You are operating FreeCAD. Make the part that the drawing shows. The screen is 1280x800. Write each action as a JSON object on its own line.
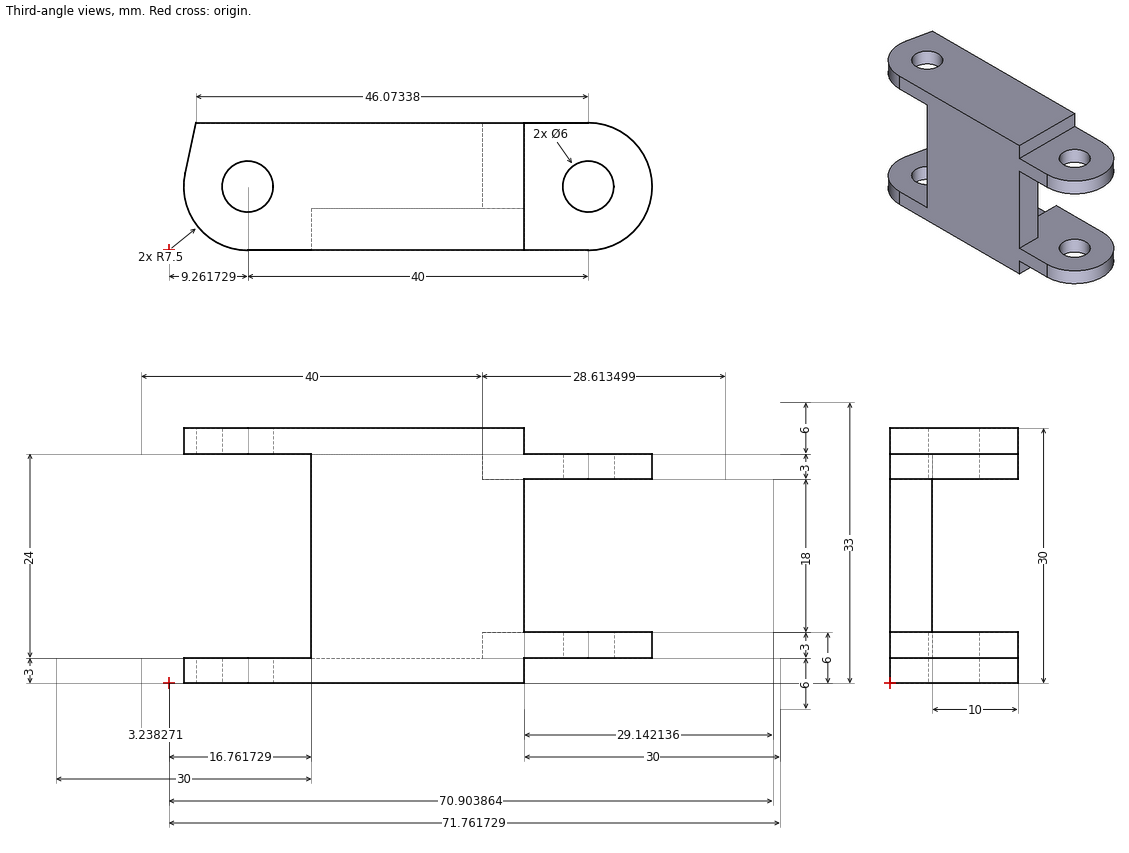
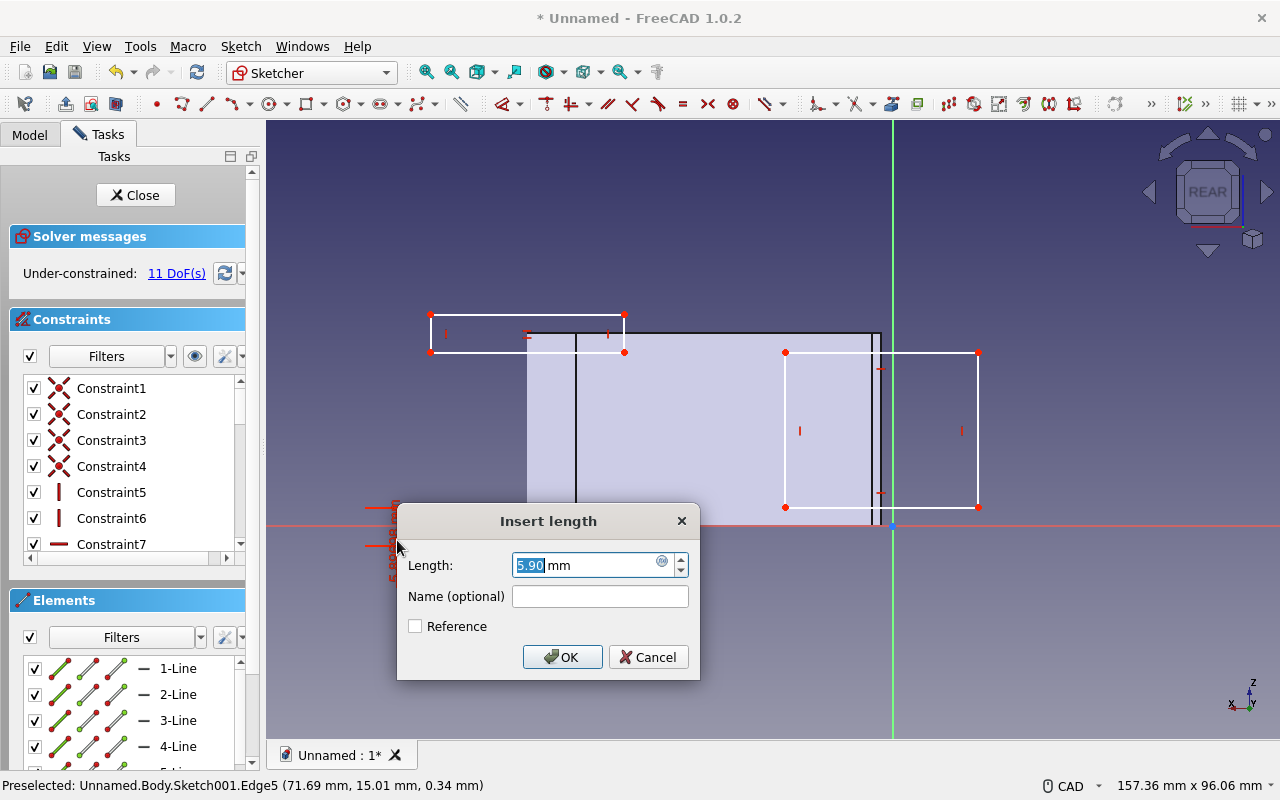
{"action": "type", "text": "6"}
{"action": "key", "text": "Return"}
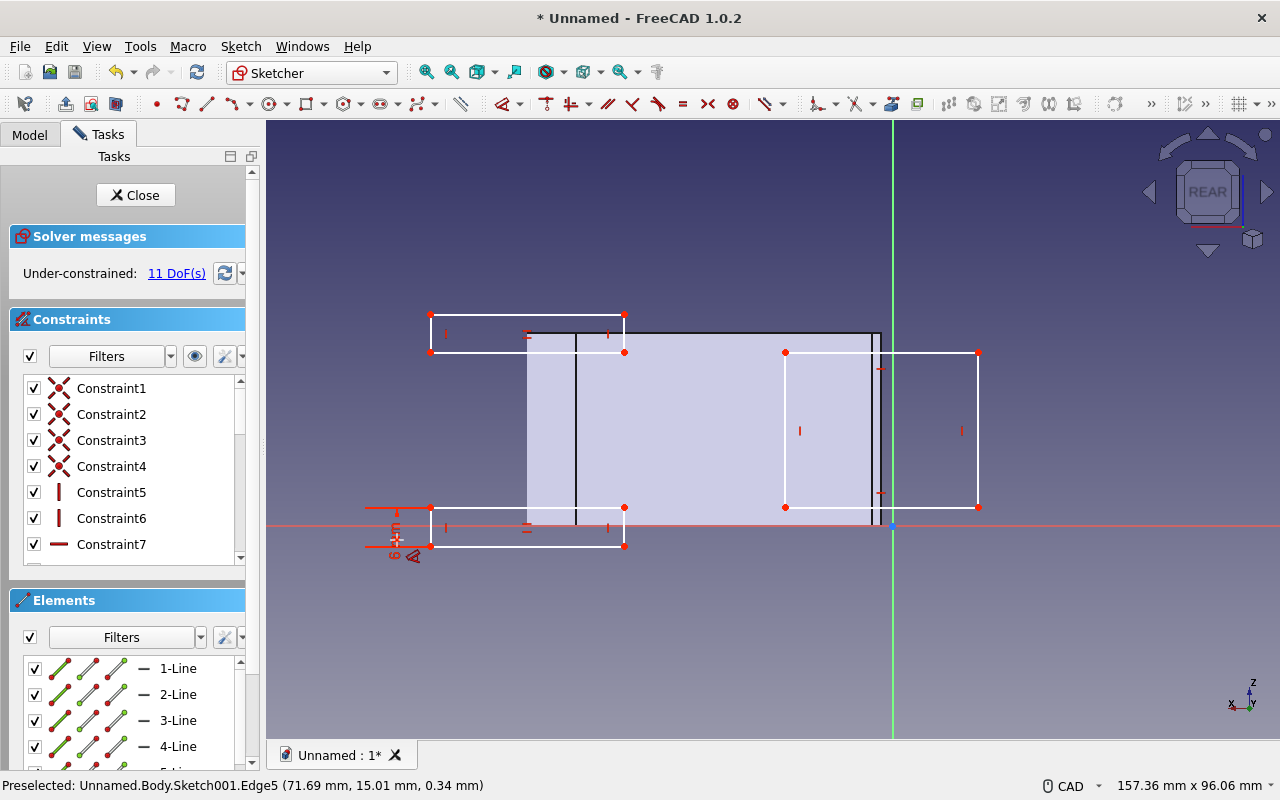
{"action": "left_click", "coordinate": [431, 326]}
{"action": "left_click", "coordinate": [397, 334]}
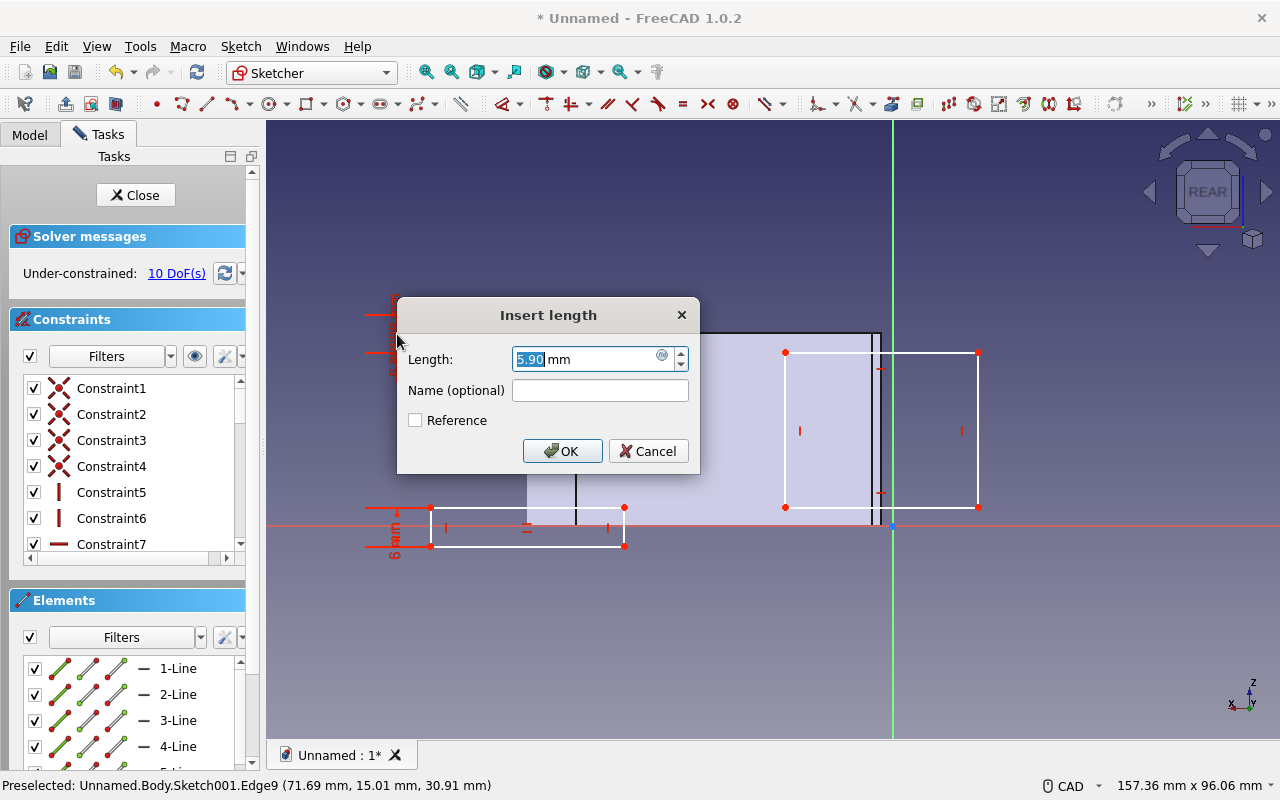
{"action": "type", "text": "6"}
{"action": "key", "text": "Return"}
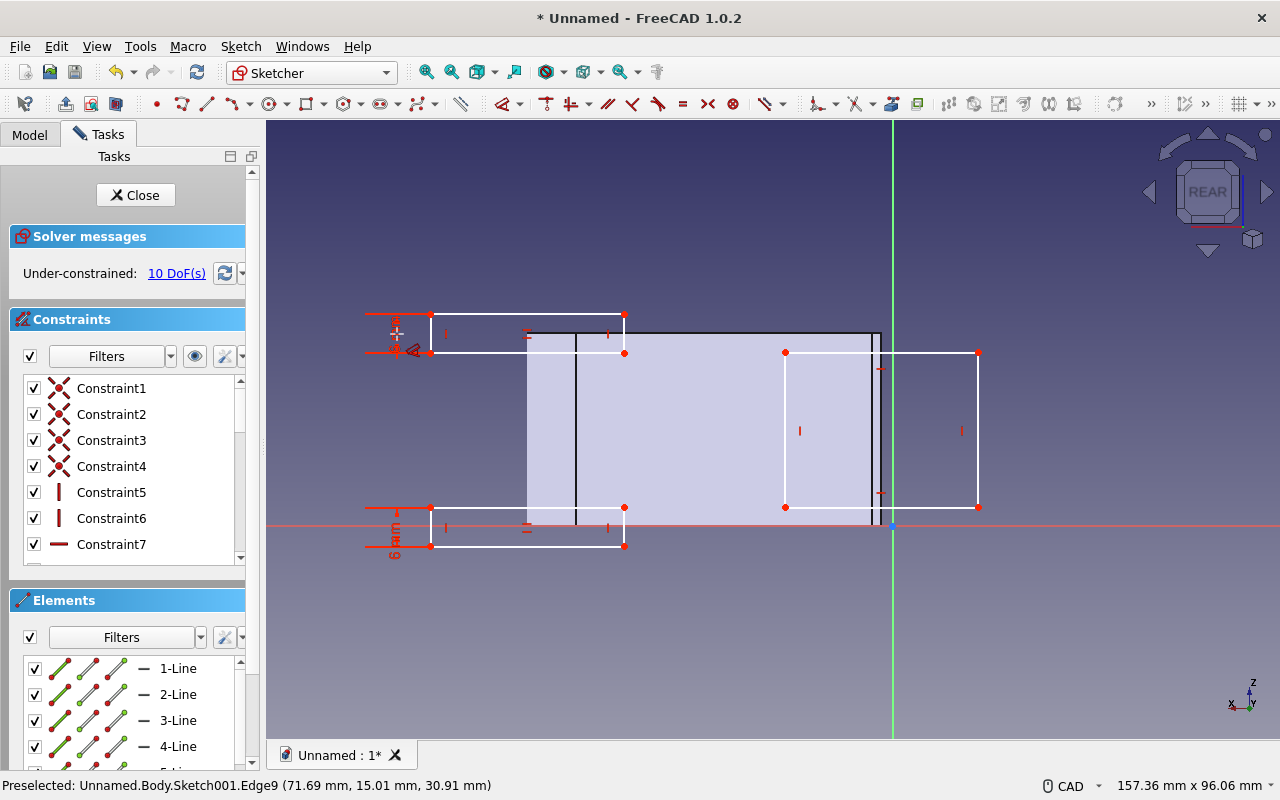
{"action": "left_click", "coordinate": [785, 399]}
{"action": "left_click", "coordinate": [819, 430]}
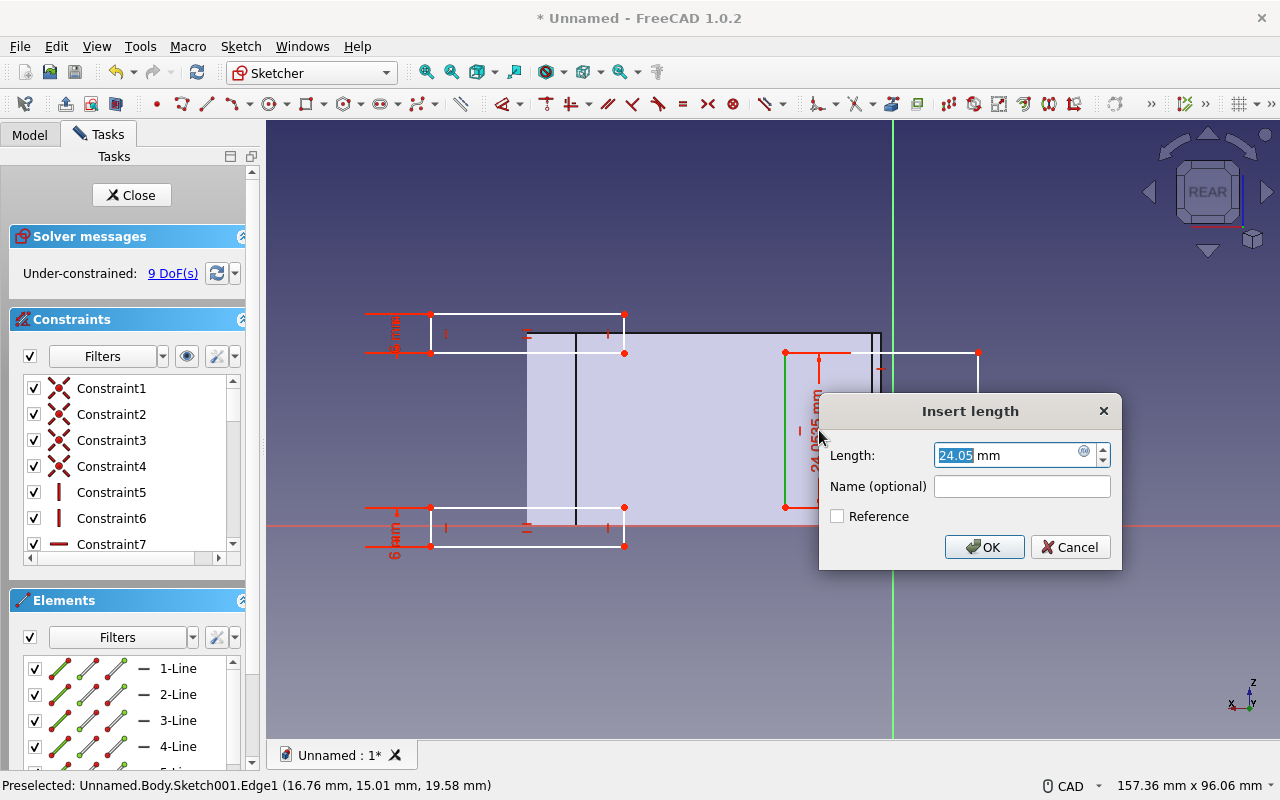
{"action": "type", "text": "24"}
{"action": "key", "text": "Return"}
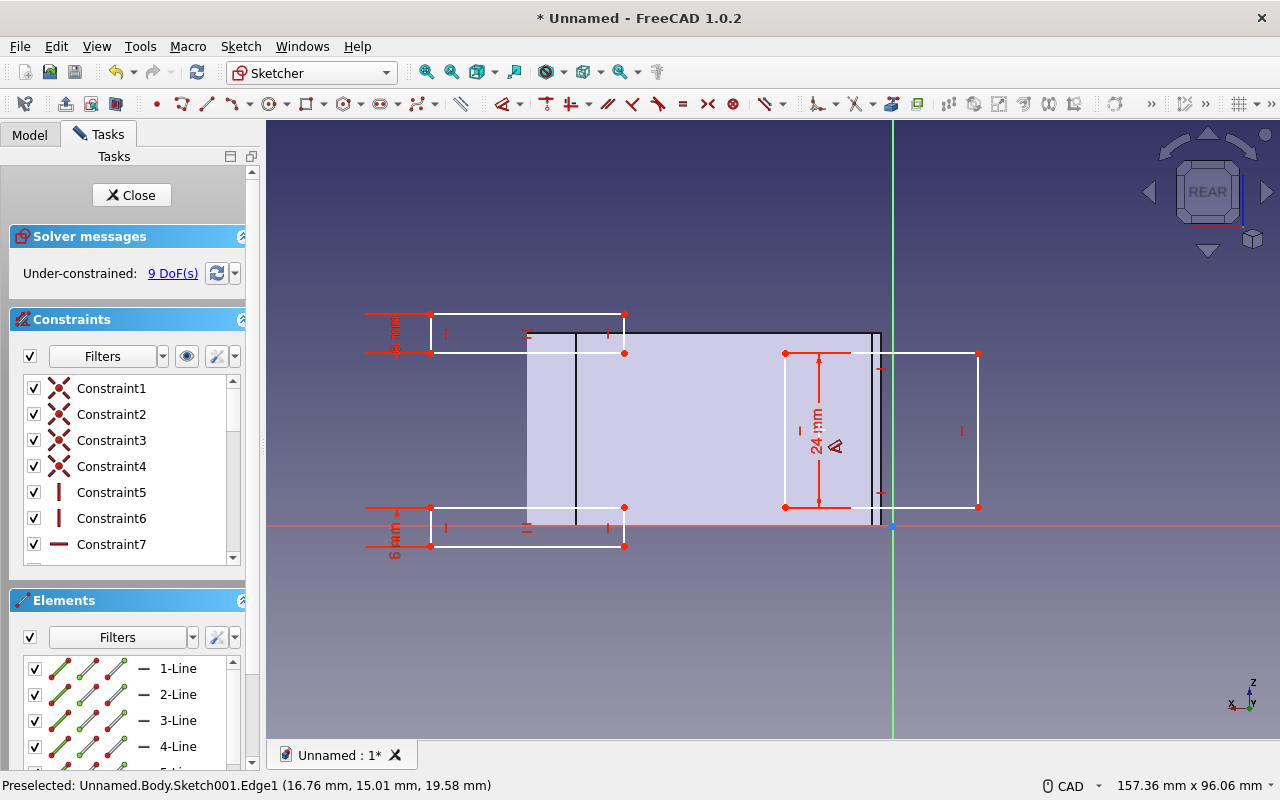
{"action": "left_click", "coordinate": [843, 508]}
{"action": "left_click", "coordinate": [837, 542]}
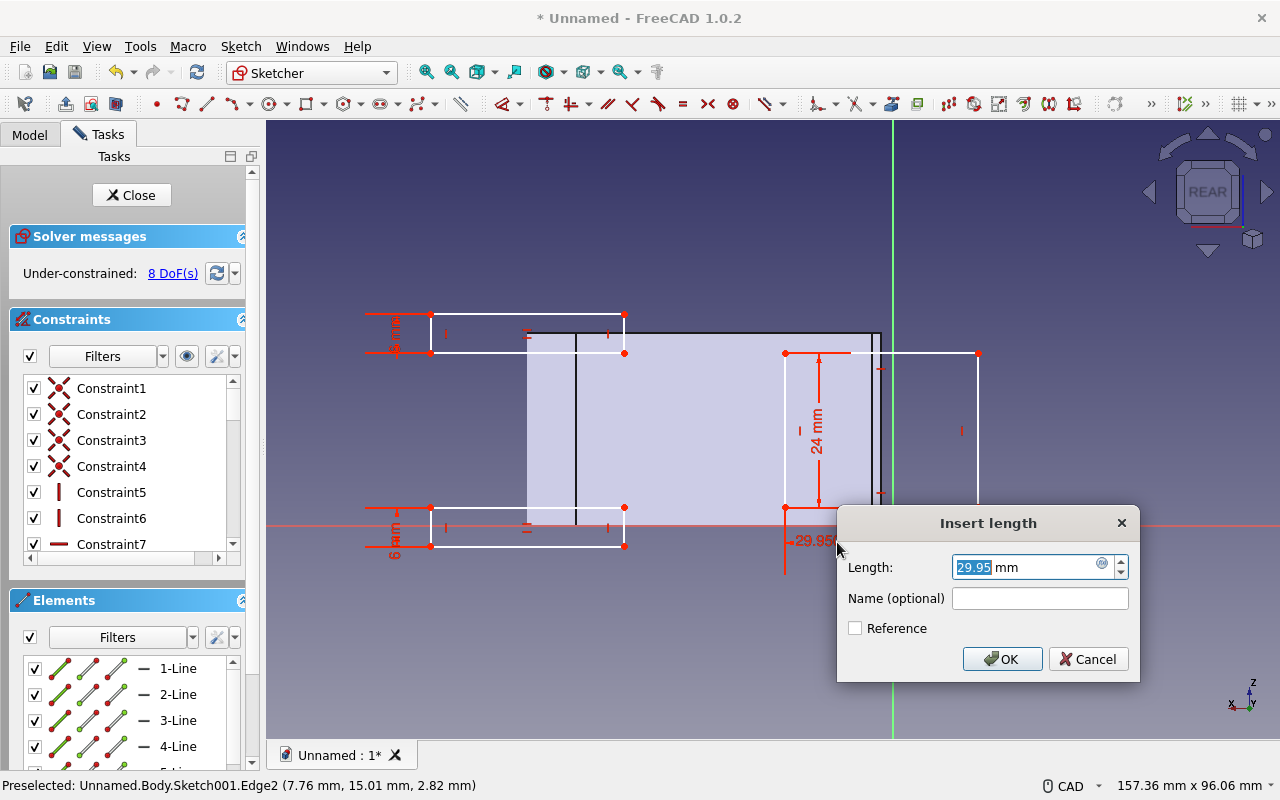
{"action": "type", "text": "30"}
{"action": "key", "text": "Return"}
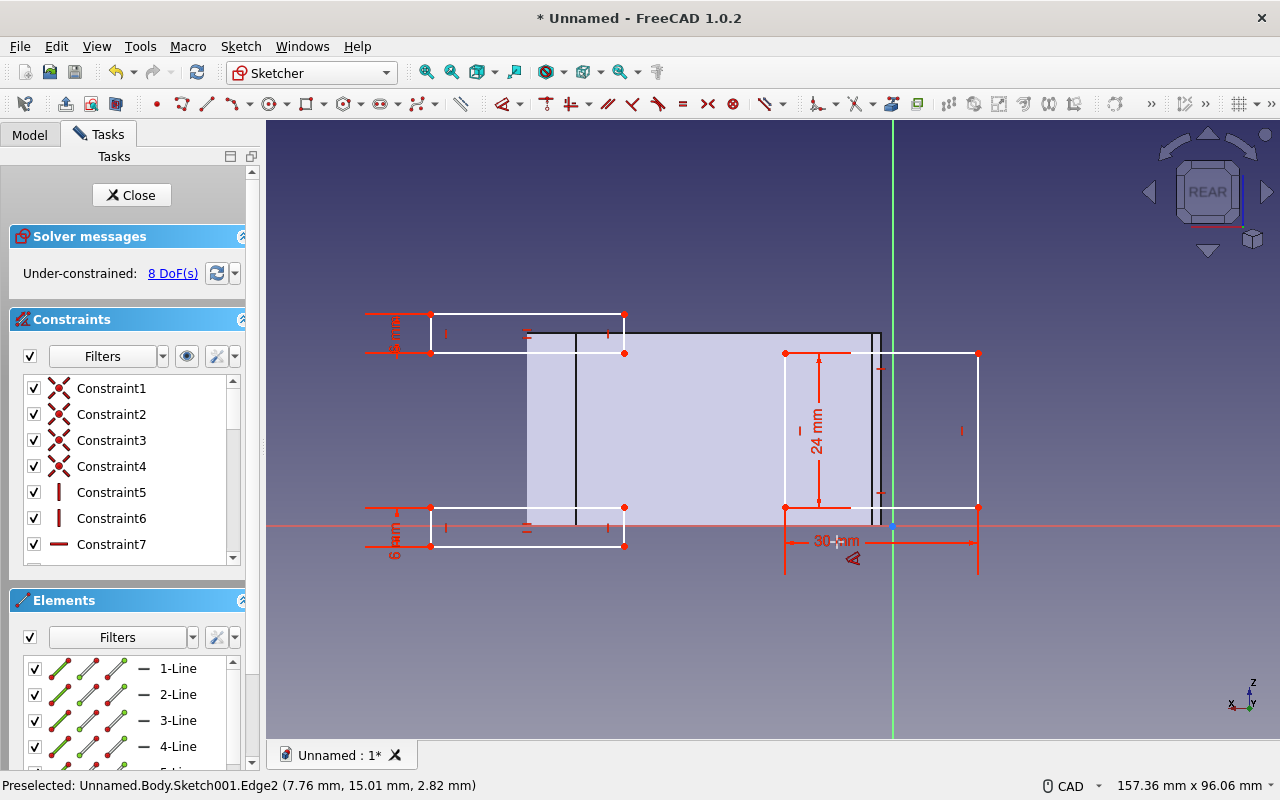
{"action": "left_click", "coordinate": [489, 547]}
{"action": "left_click", "coordinate": [528, 581]}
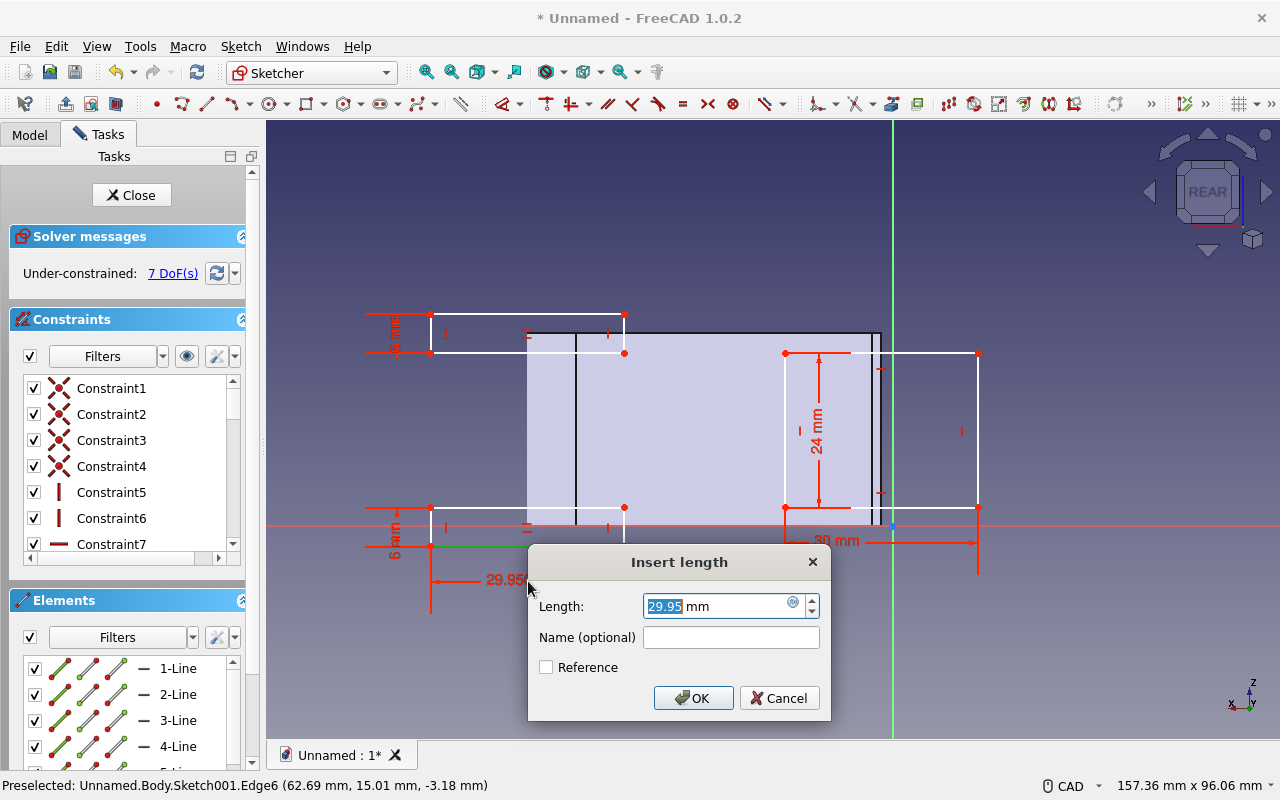
{"action": "type", "text": "30"}
{"action": "key", "text": "Return"}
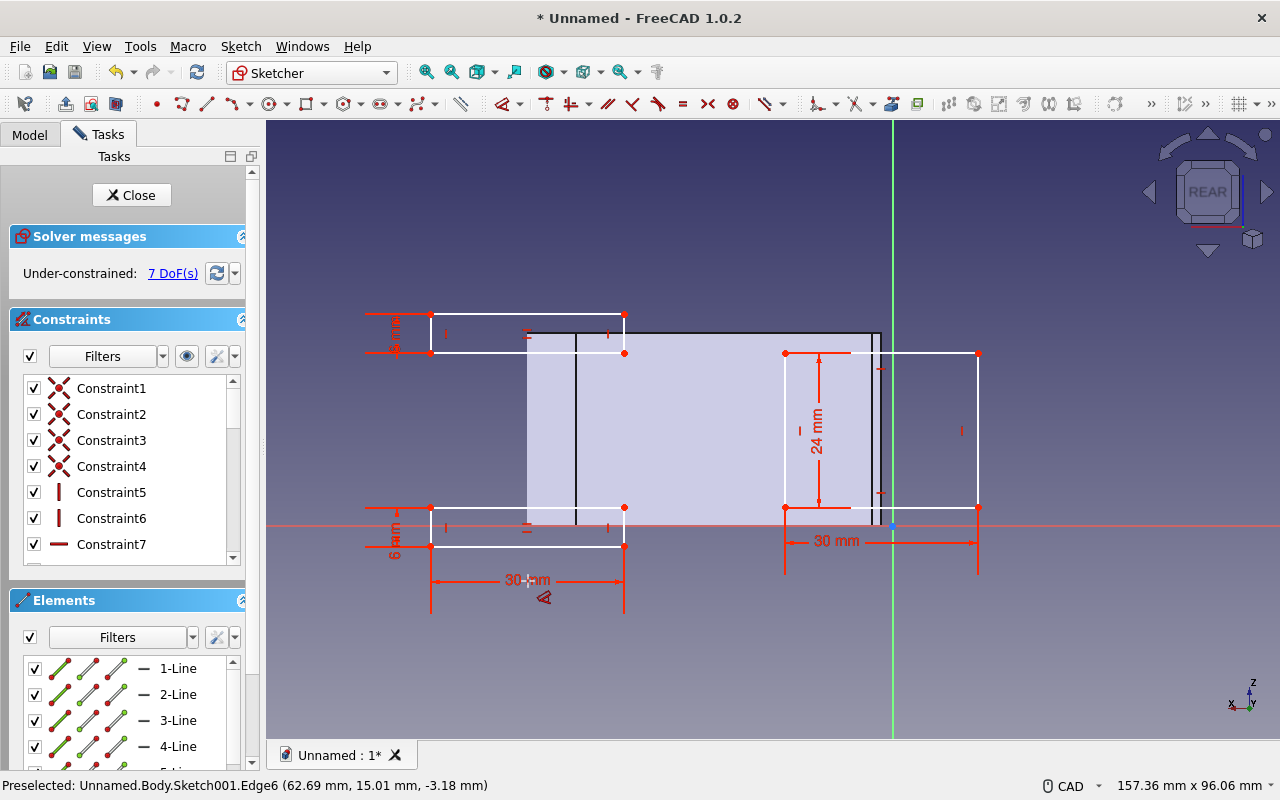
{"action": "left_click", "coordinate": [489, 353]}
{"action": "left_click", "coordinate": [528, 387]}